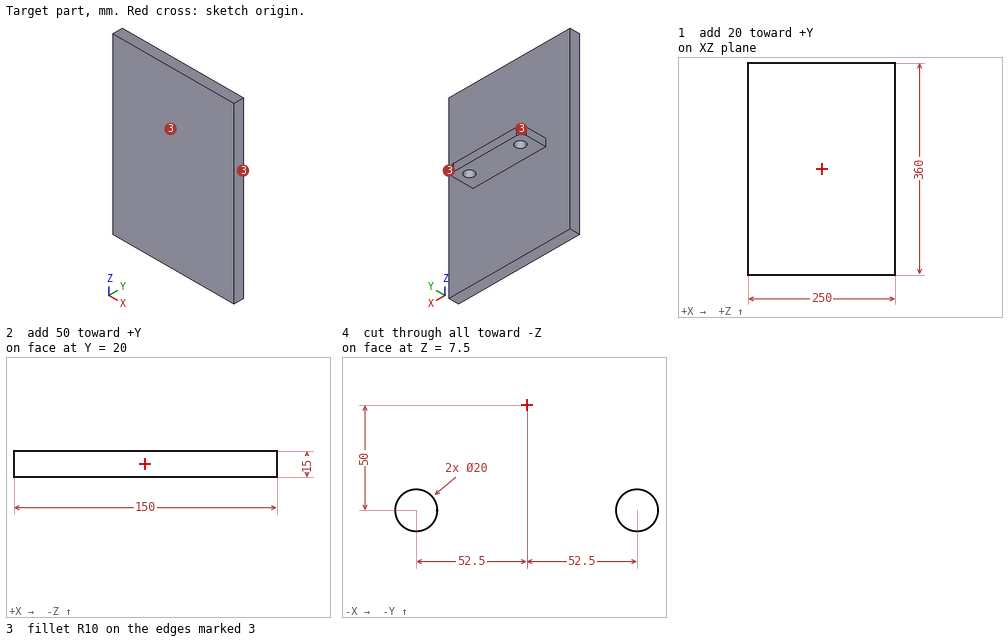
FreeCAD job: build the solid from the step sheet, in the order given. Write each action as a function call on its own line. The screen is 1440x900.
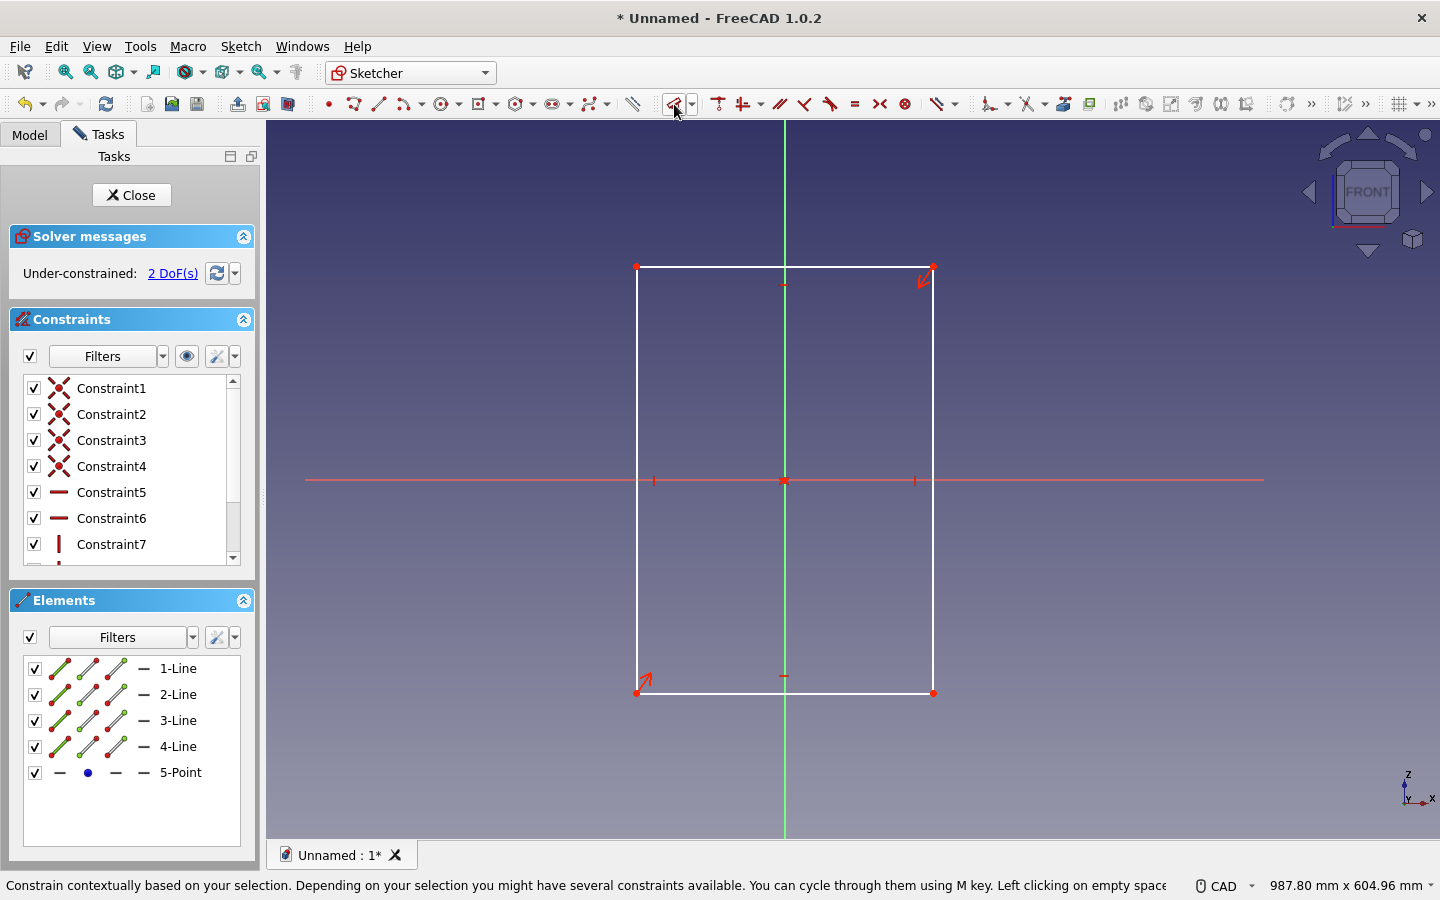
click(726, 694)
click(717, 728)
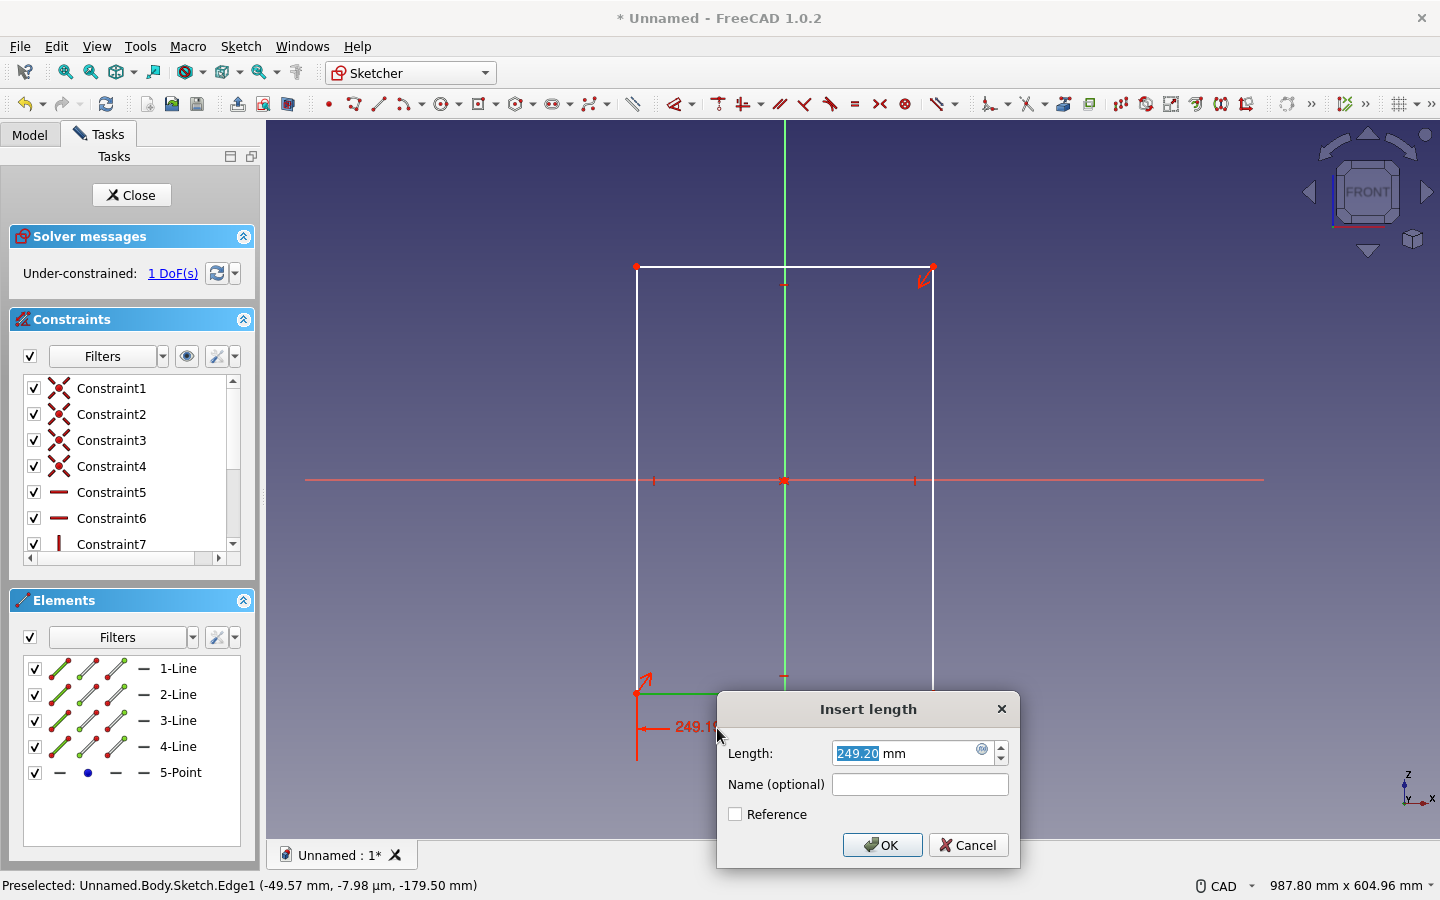
text(250)
key(Return)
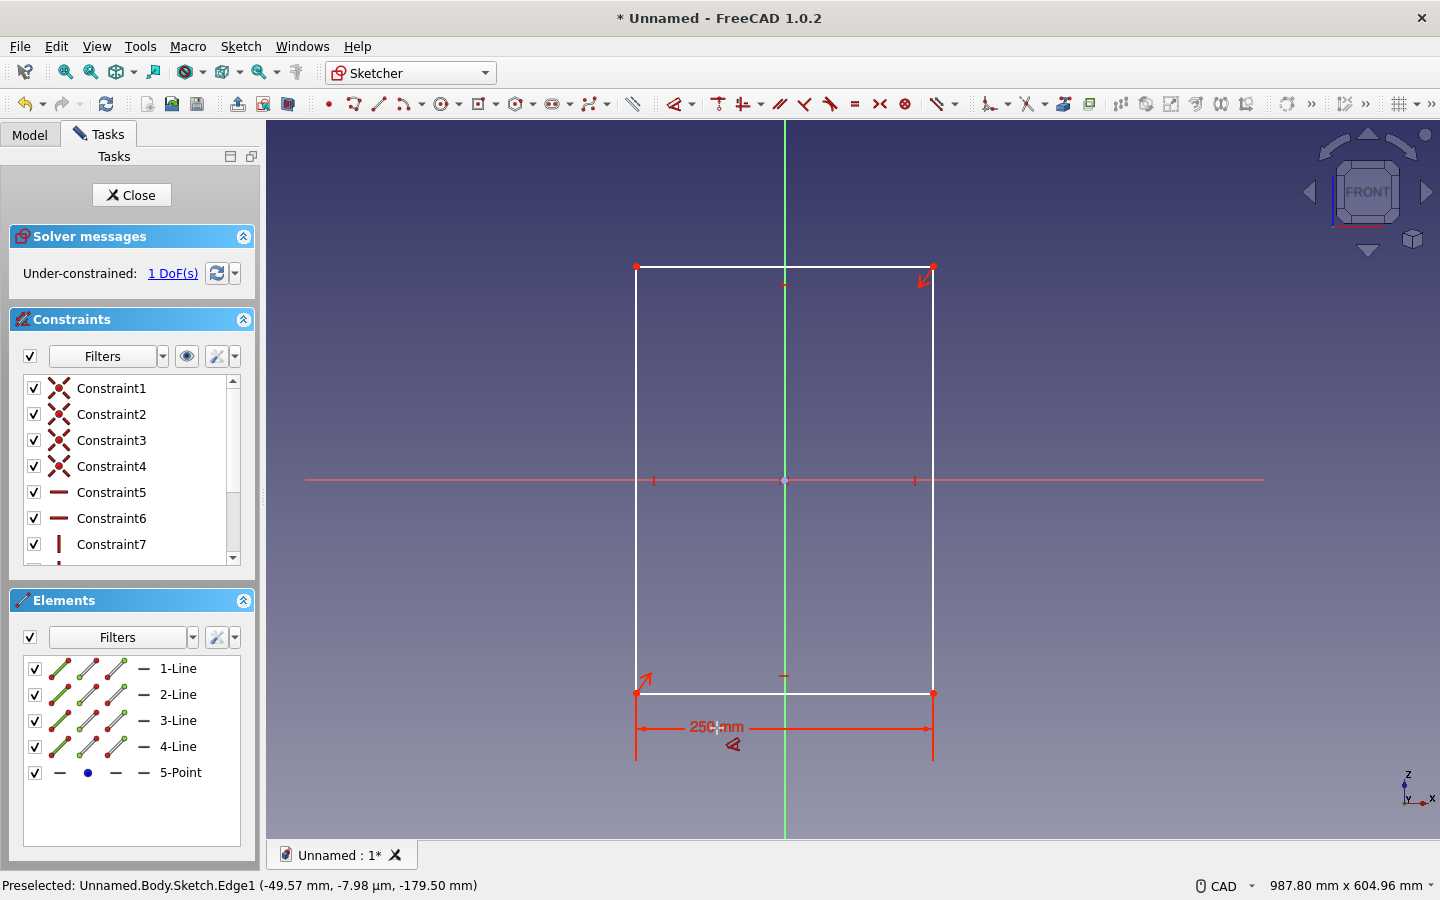
click(933, 566)
click(967, 382)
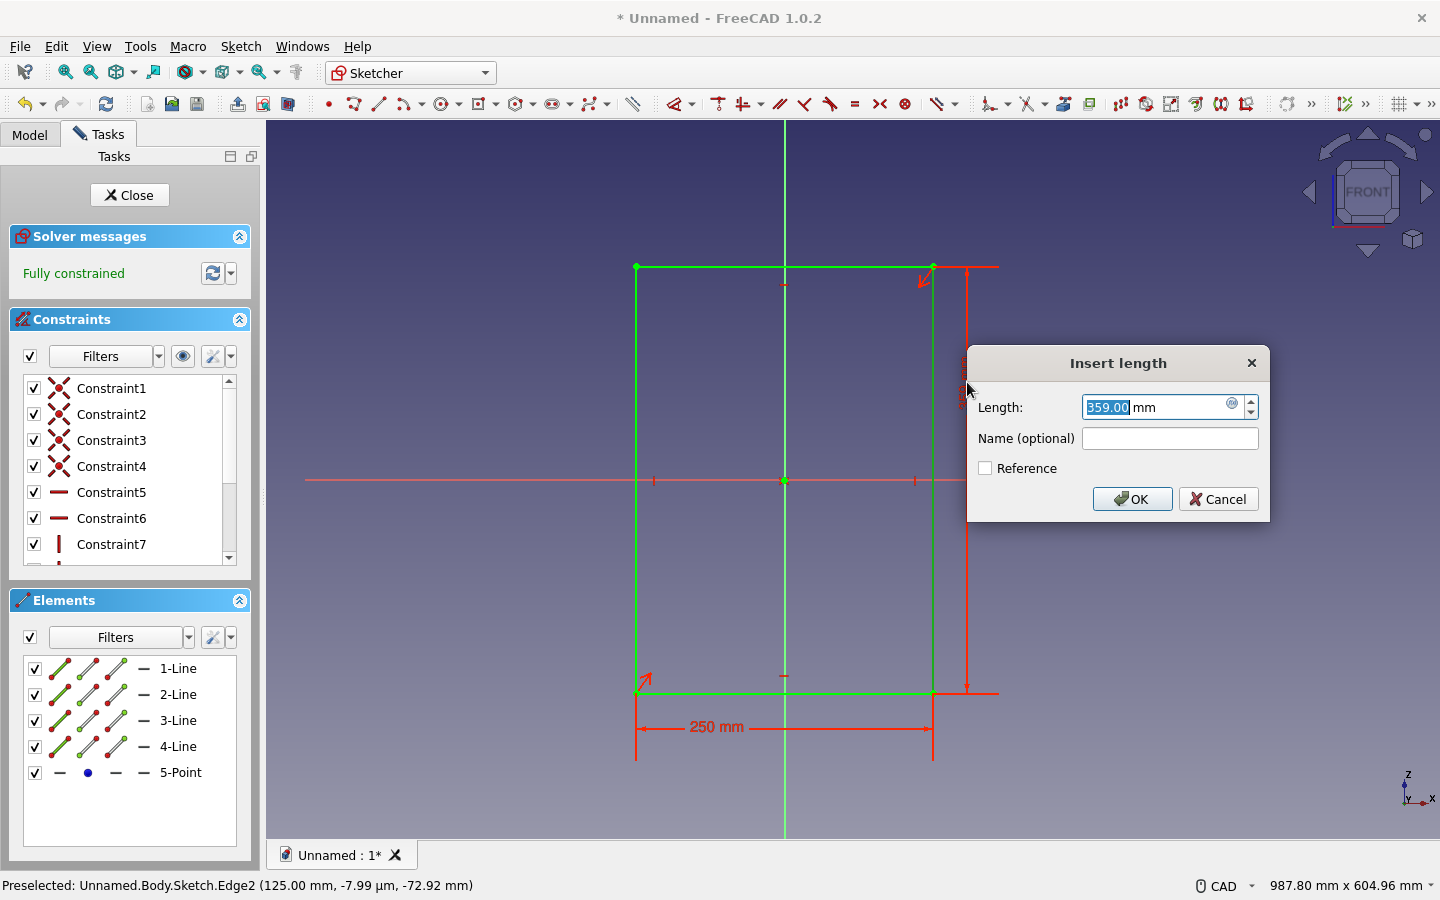
text(360)
key(Return)
key(Escape)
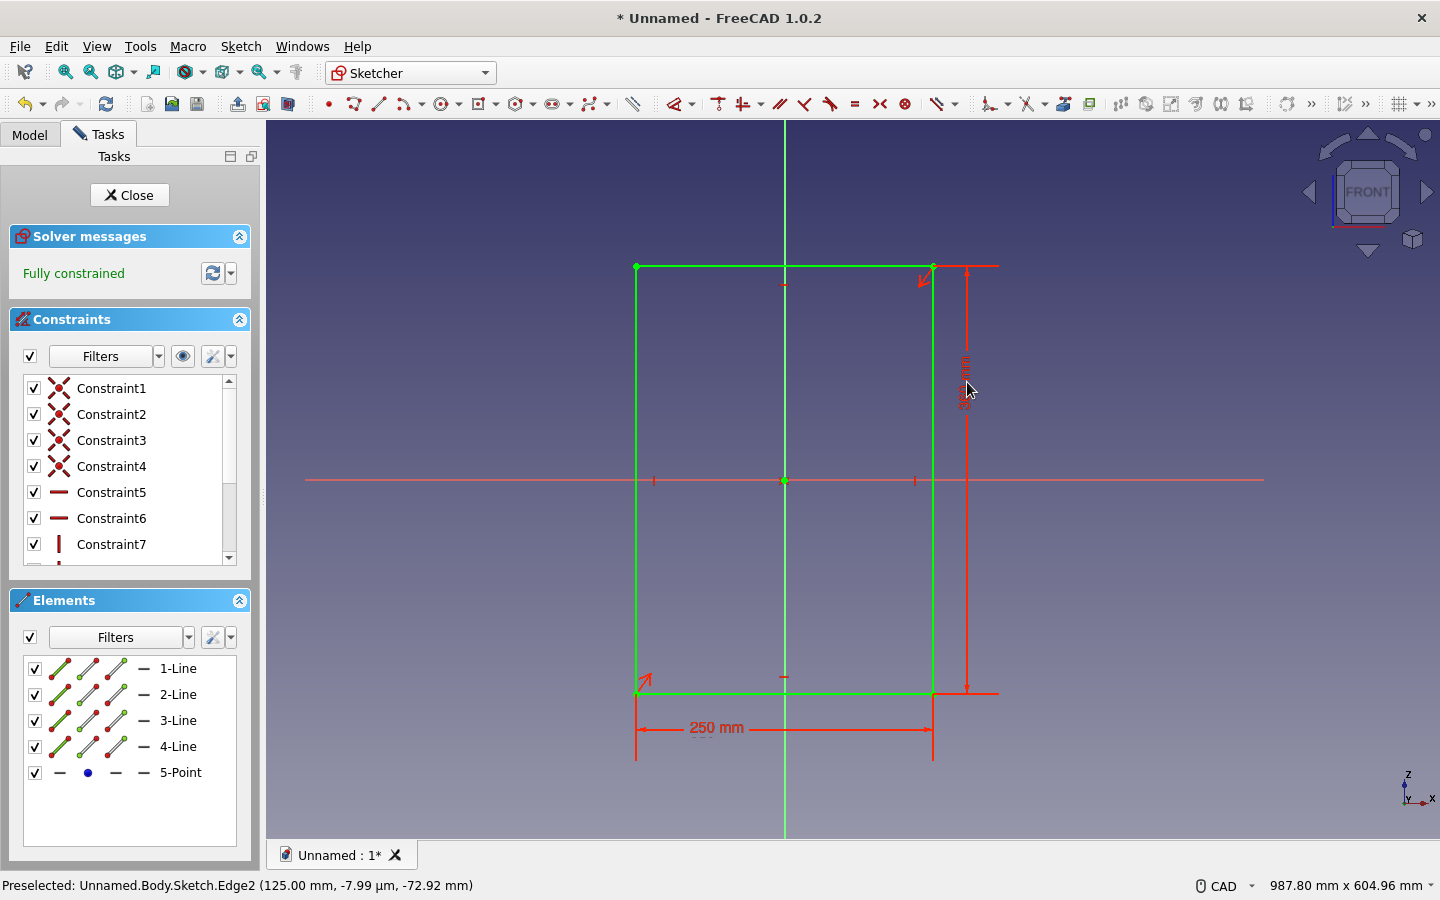
click(130, 195)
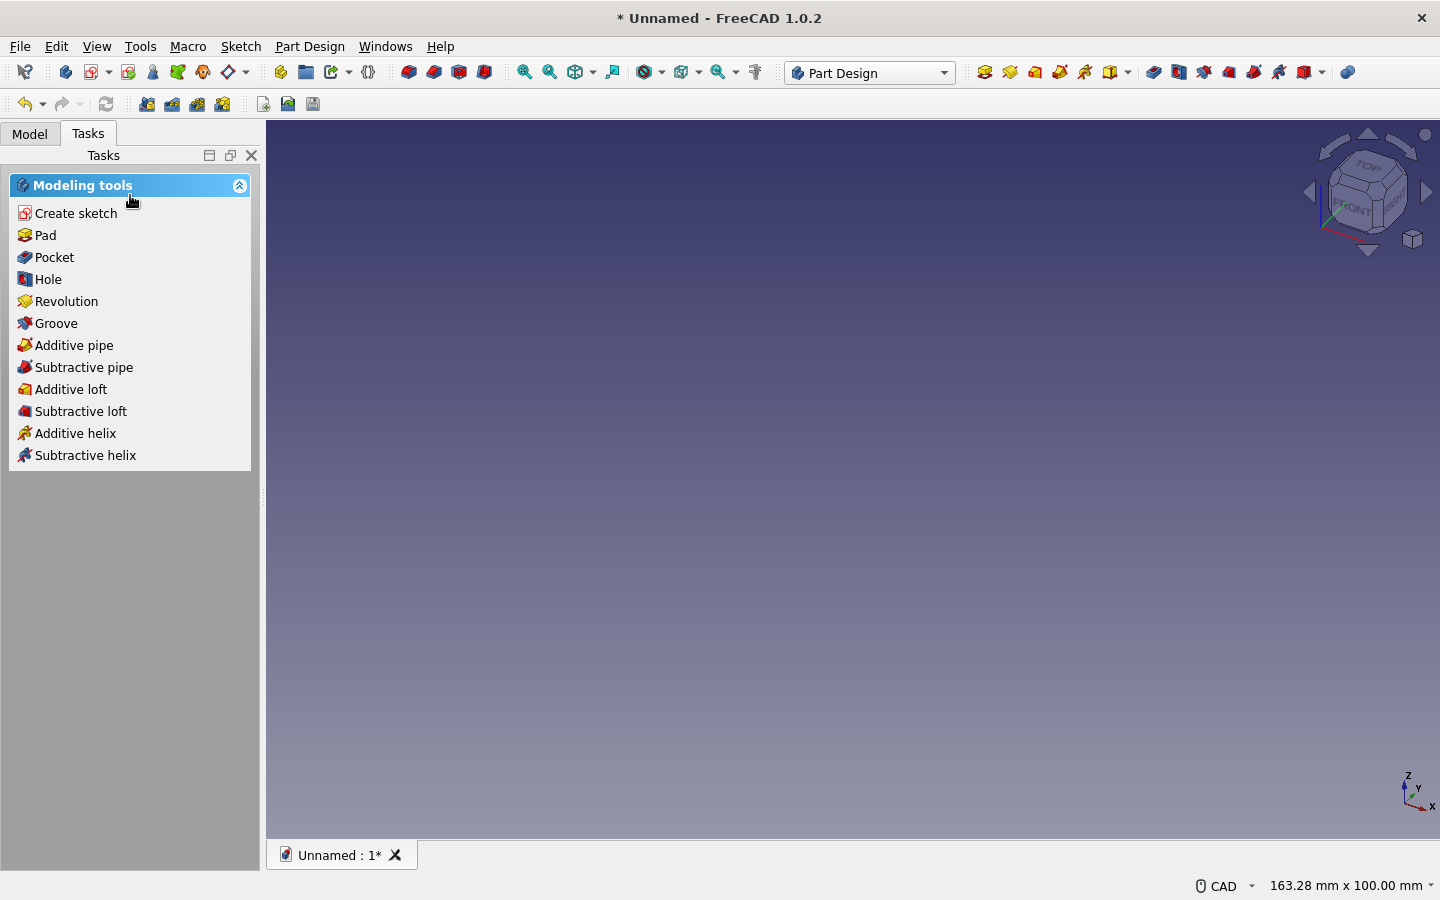
click(985, 72)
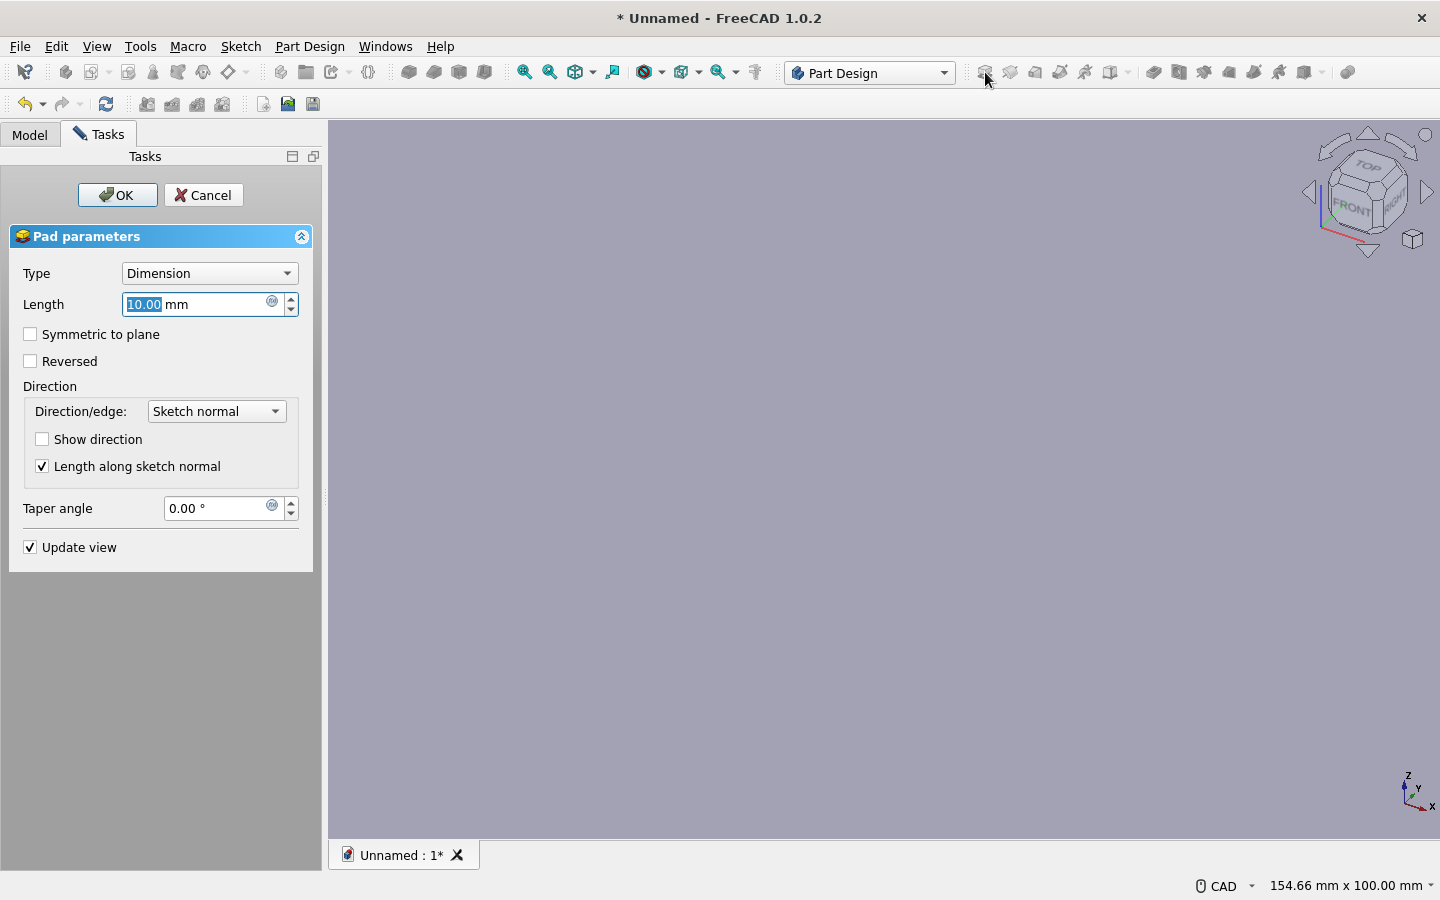
text(20)
key(Tab)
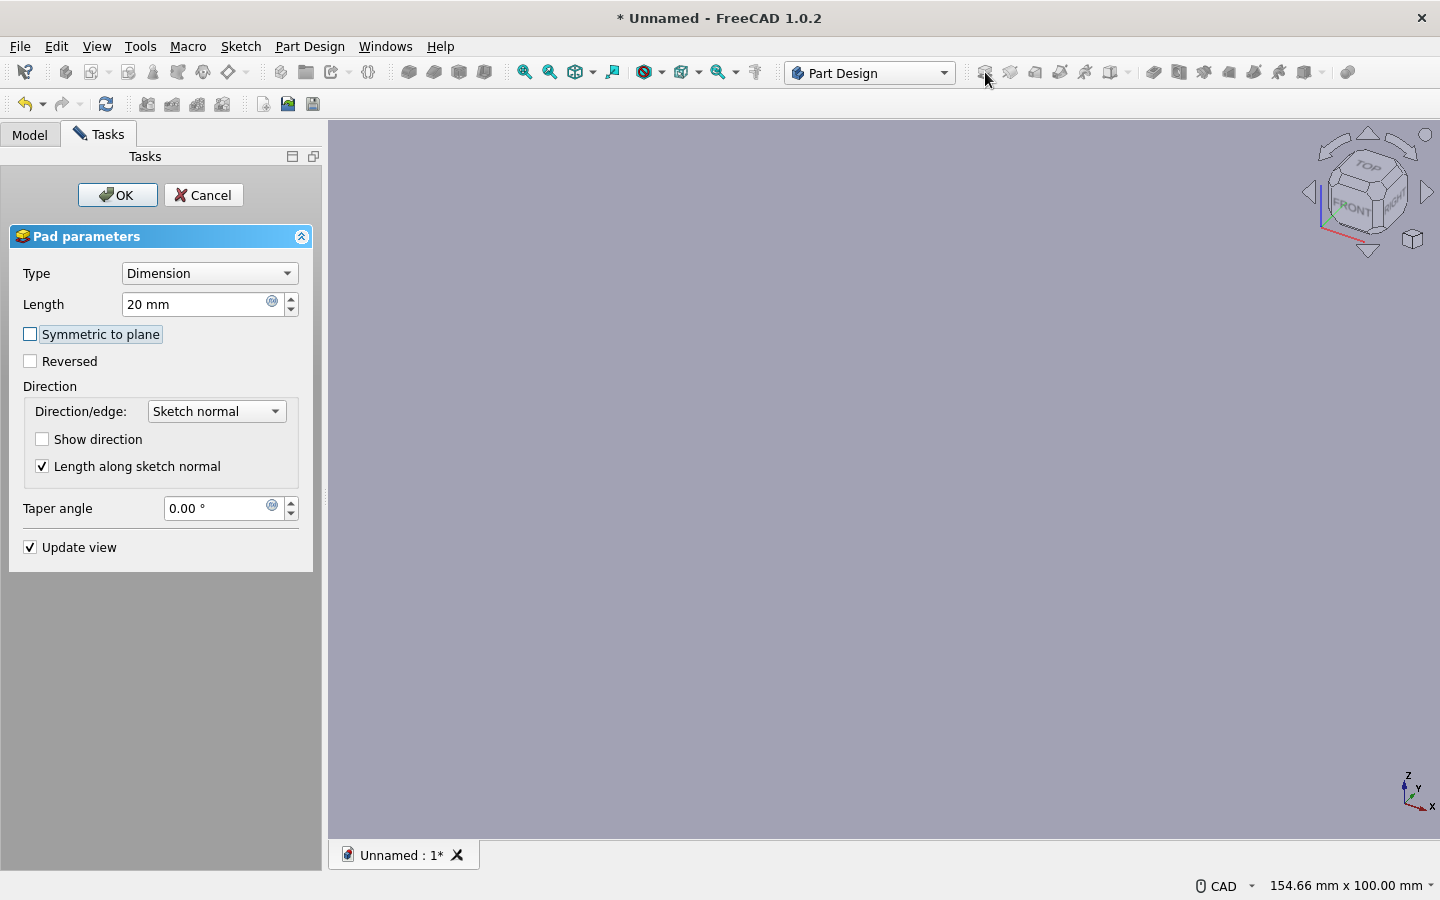
click(31, 361)